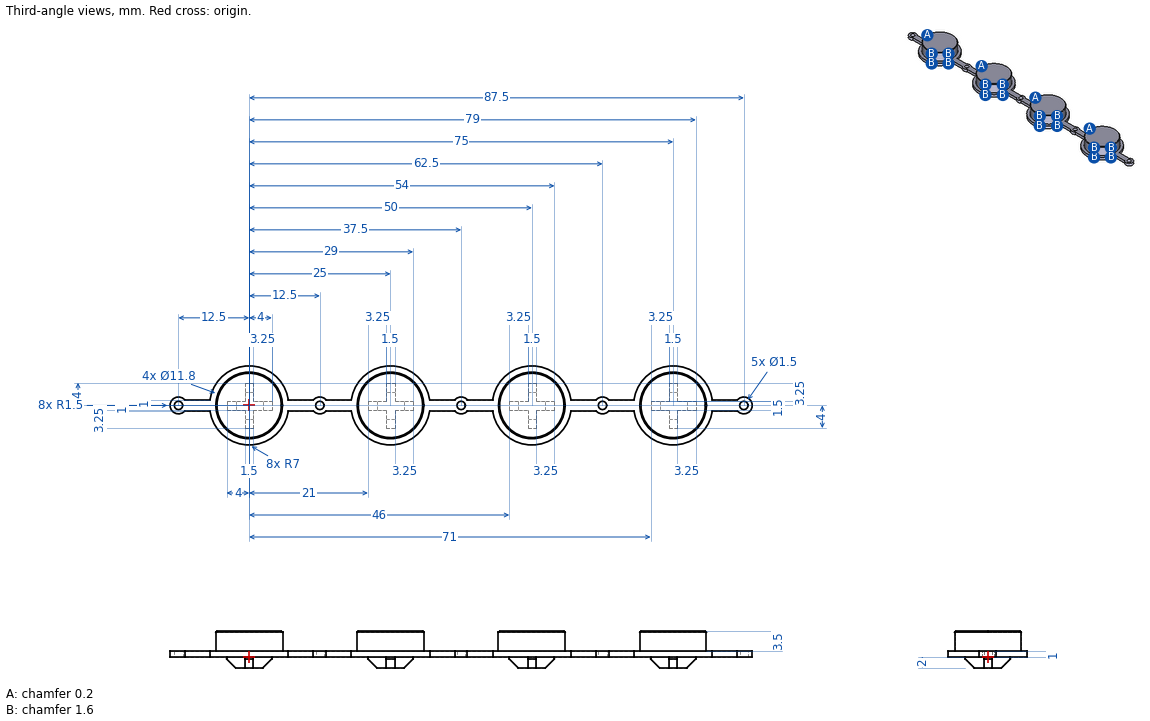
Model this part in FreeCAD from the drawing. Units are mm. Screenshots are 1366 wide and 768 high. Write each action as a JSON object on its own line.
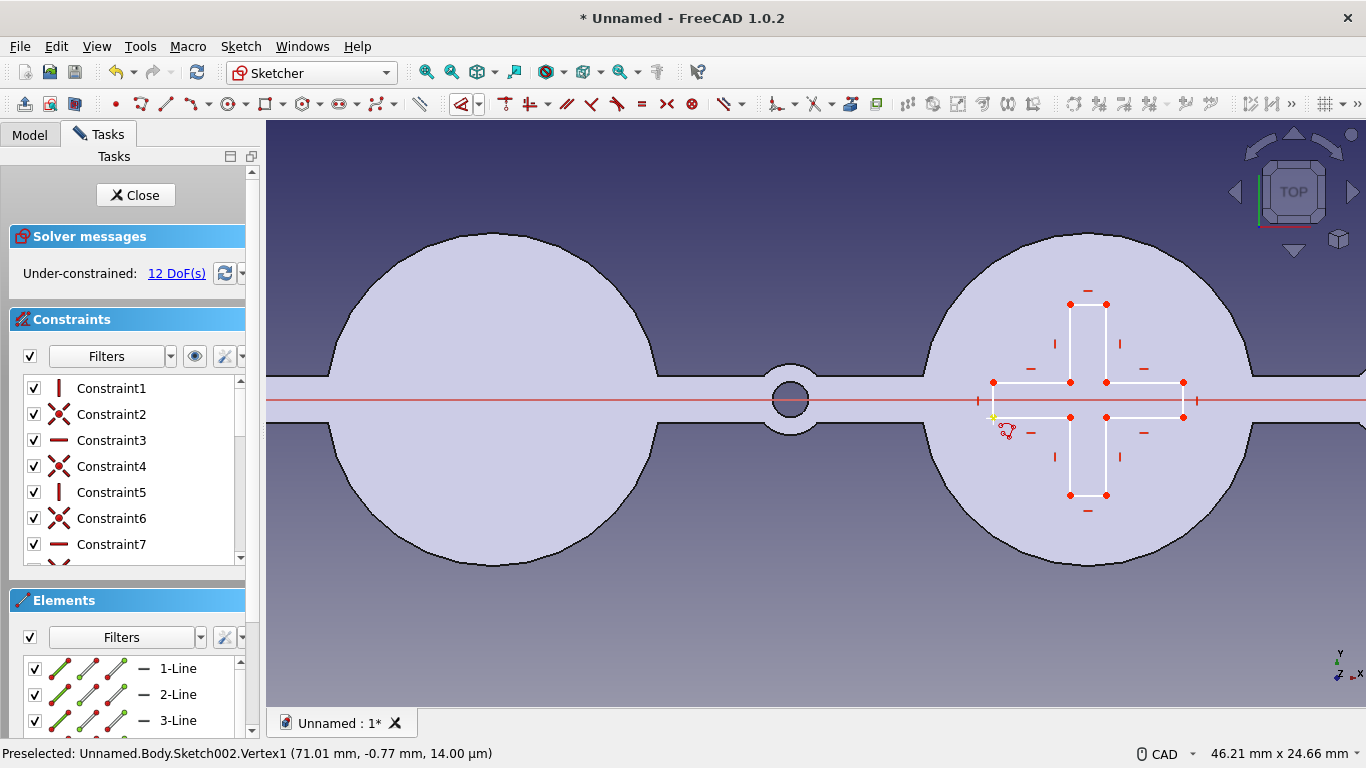
{"action": "left_click", "coordinate": [398, 417]}
{"action": "left_click", "coordinate": [398, 382]}
{"action": "left_click", "coordinate": [475, 382]}
{"action": "left_click", "coordinate": [475, 304]}
{"action": "left_click", "coordinate": [511, 304]}
{"action": "left_click", "coordinate": [511, 382]}
{"action": "left_click", "coordinate": [588, 382]}
{"action": "left_click", "coordinate": [588, 417]}
{"action": "left_click", "coordinate": [511, 417]}
{"action": "left_click", "coordinate": [511, 495]}
{"action": "left_click", "coordinate": [475, 495]}
{"action": "left_click", "coordinate": [475, 417]}
{"action": "left_click", "coordinate": [398, 418]}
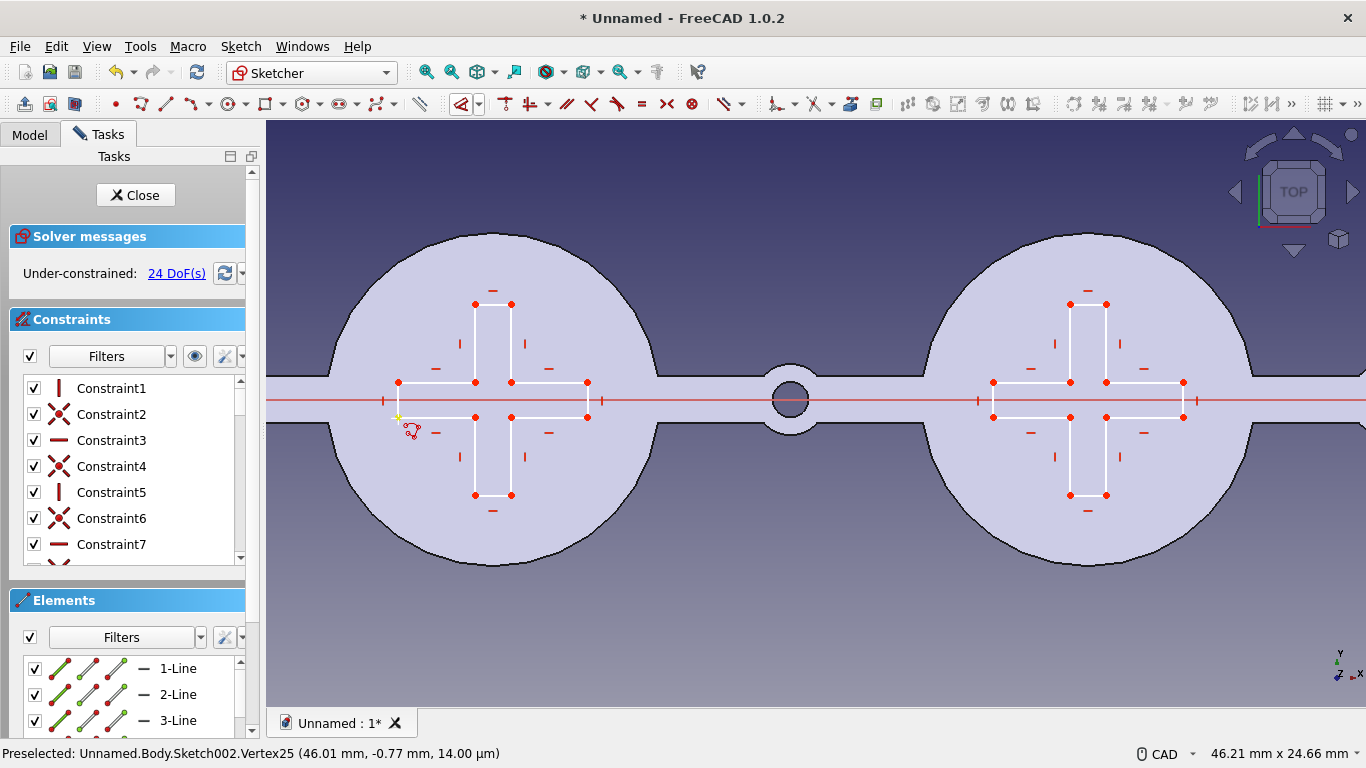
{"action": "scroll", "coordinate": [985, 420], "scroll_direction": "down", "scroll_amount": 6}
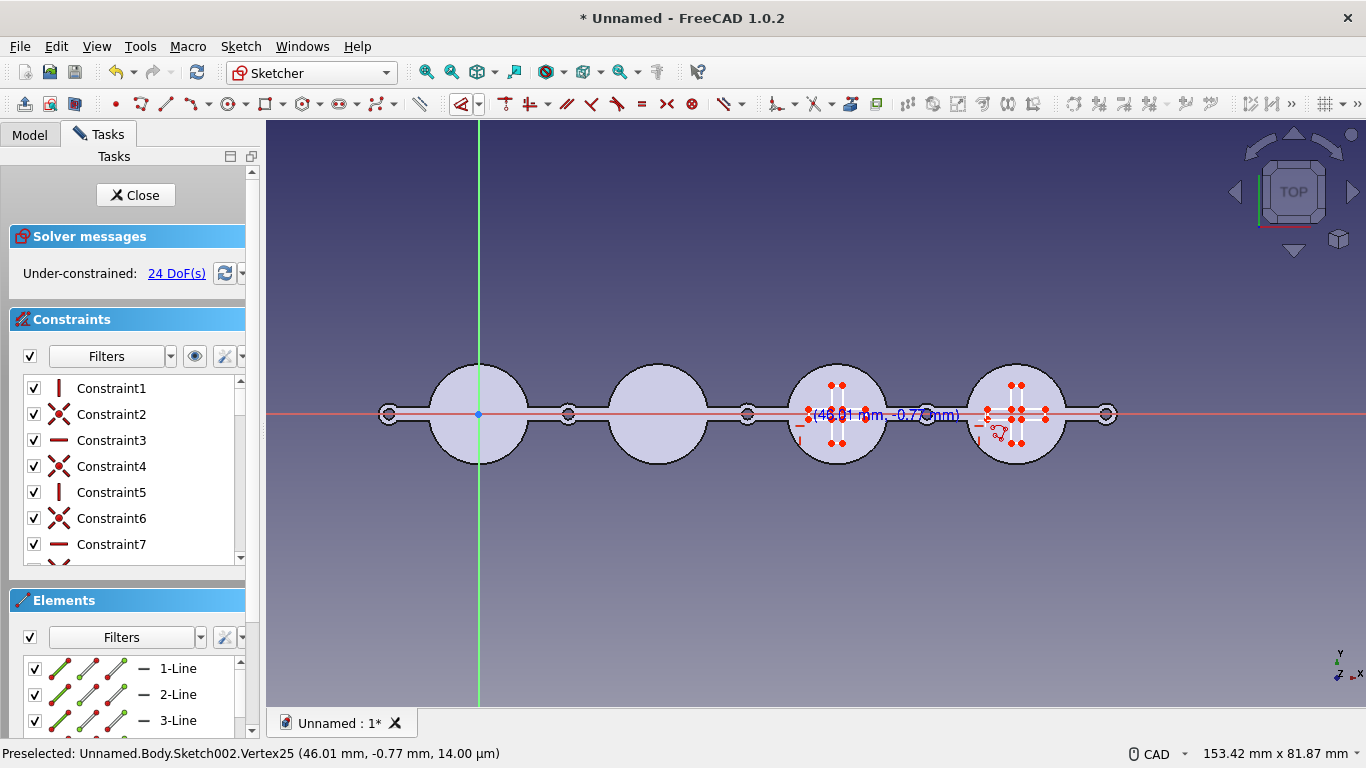
{"action": "scroll", "coordinate": [629, 420], "scroll_direction": "up", "scroll_amount": 6}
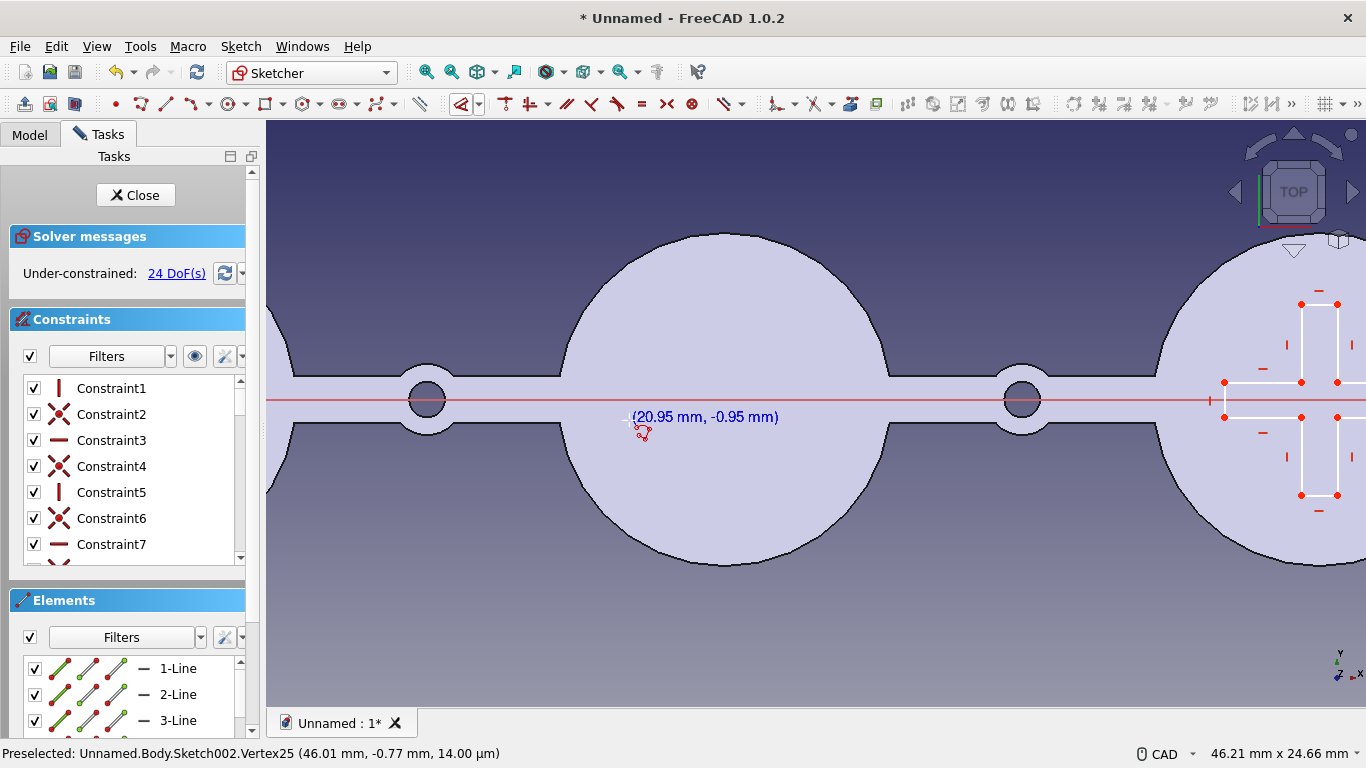
{"action": "left_click", "coordinate": [629, 417]}
{"action": "left_click", "coordinate": [629, 382]}
{"action": "left_click", "coordinate": [707, 382]}
{"action": "left_click", "coordinate": [707, 304]}
{"action": "left_click", "coordinate": [742, 304]}
{"action": "left_click", "coordinate": [742, 382]}
{"action": "left_click", "coordinate": [820, 382]}
{"action": "left_click", "coordinate": [820, 417]}
{"action": "left_click", "coordinate": [742, 417]}
{"action": "left_click", "coordinate": [742, 495]}
{"action": "left_click", "coordinate": [707, 495]}
{"action": "left_click", "coordinate": [707, 417]}
{"action": "left_click", "coordinate": [629, 418]}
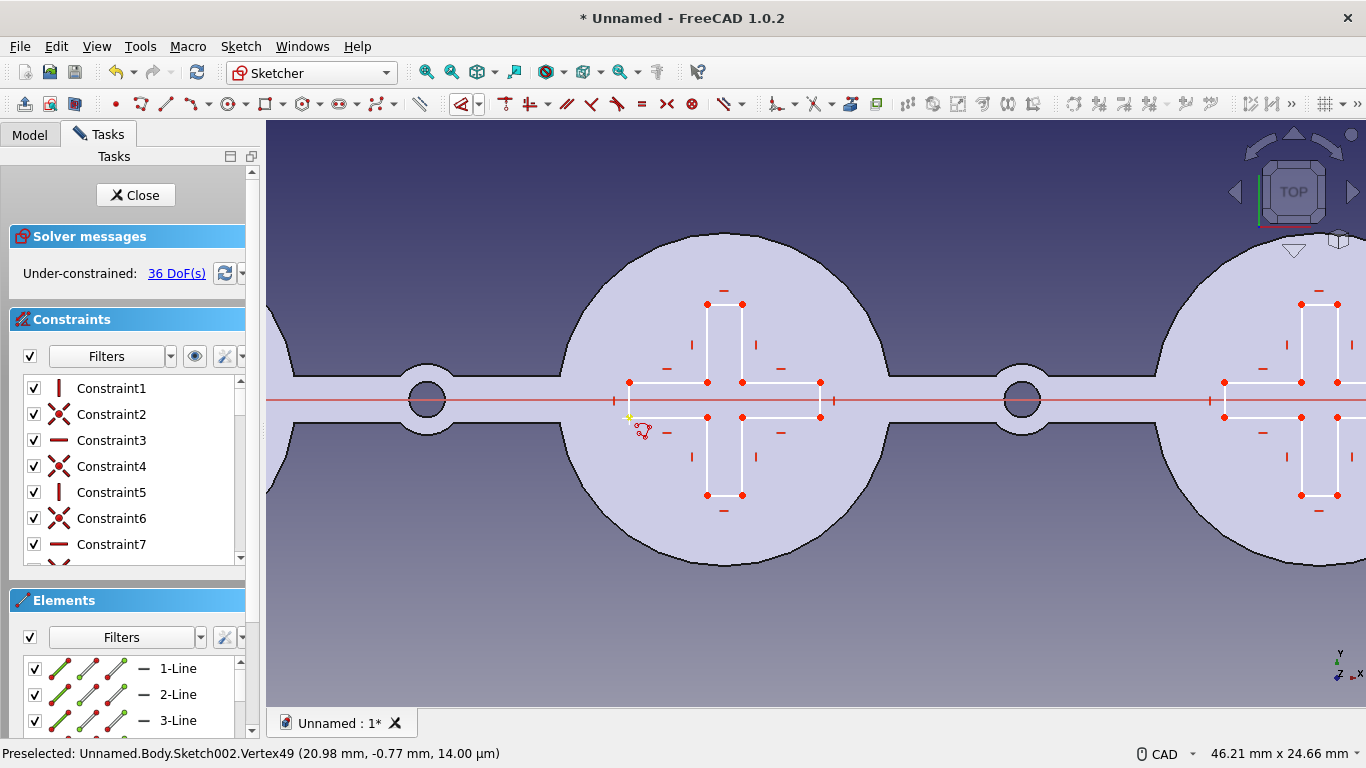
{"action": "scroll", "coordinate": [629, 420], "scroll_direction": "down", "scroll_amount": 6}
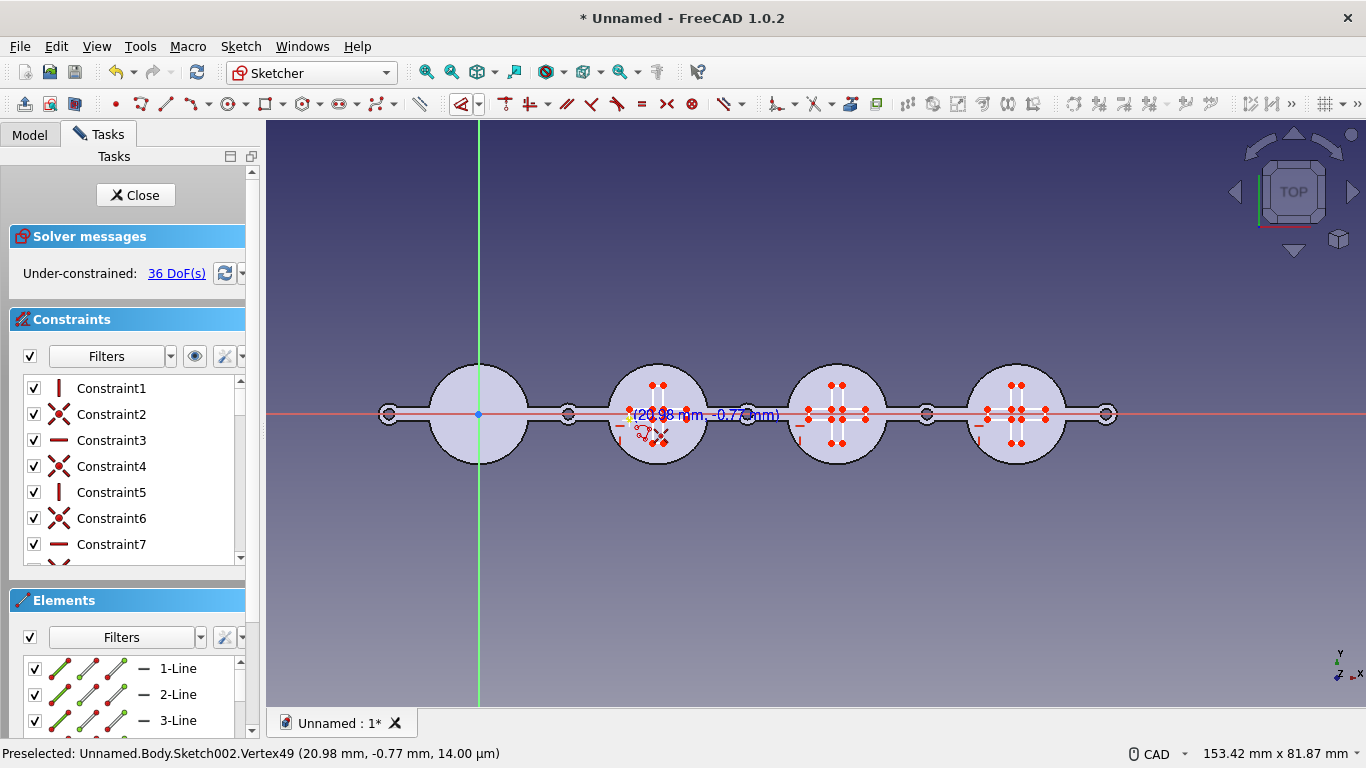
{"action": "scroll", "coordinate": [484, 409], "scroll_direction": "up", "scroll_amount": 6}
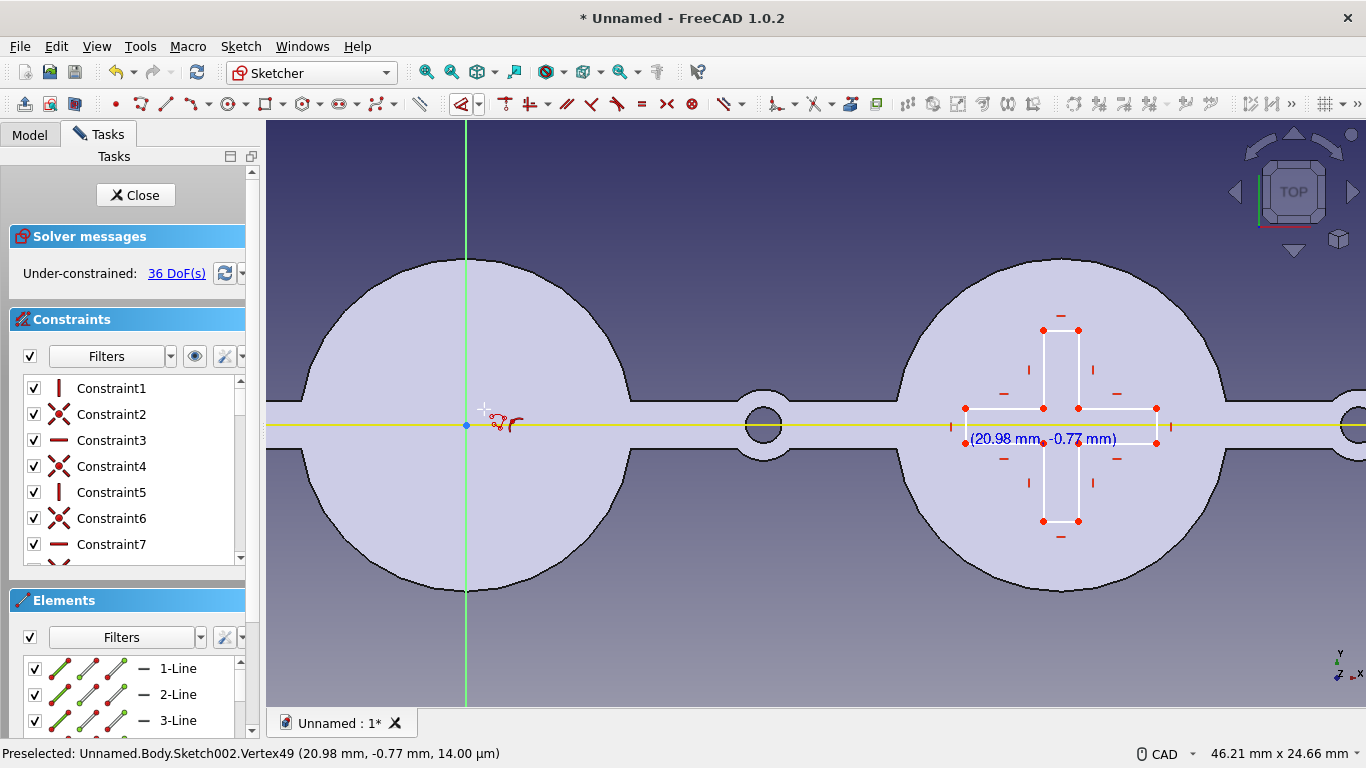
{"action": "left_click", "coordinate": [484, 407]}
{"action": "left_click", "coordinate": [561, 407]}
{"action": "left_click", "coordinate": [561, 443]}
{"action": "left_click", "coordinate": [484, 443]}
{"action": "left_click", "coordinate": [484, 520]}
{"action": "left_click", "coordinate": [448, 520]}
{"action": "left_click", "coordinate": [448, 443]}
{"action": "left_click", "coordinate": [371, 443]}
{"action": "left_click", "coordinate": [371, 407]}
{"action": "left_click", "coordinate": [448, 407]}
{"action": "left_click", "coordinate": [448, 330]}
{"action": "left_click", "coordinate": [484, 330]}
{"action": "left_click", "coordinate": [484, 408]}
{"action": "key", "text": "Escape"}
{"action": "key", "text": "Escape"}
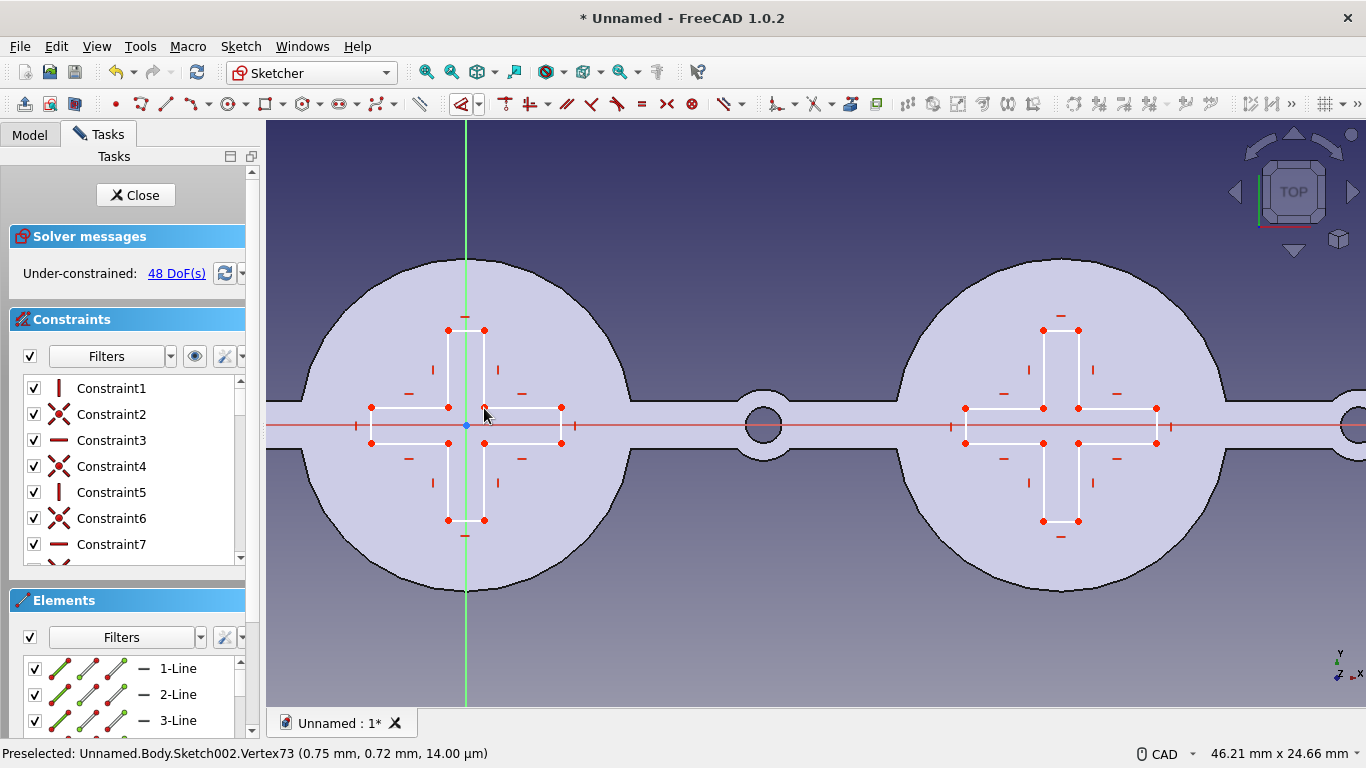
{"action": "scroll", "coordinate": [484, 408], "scroll_direction": "down", "scroll_amount": 6}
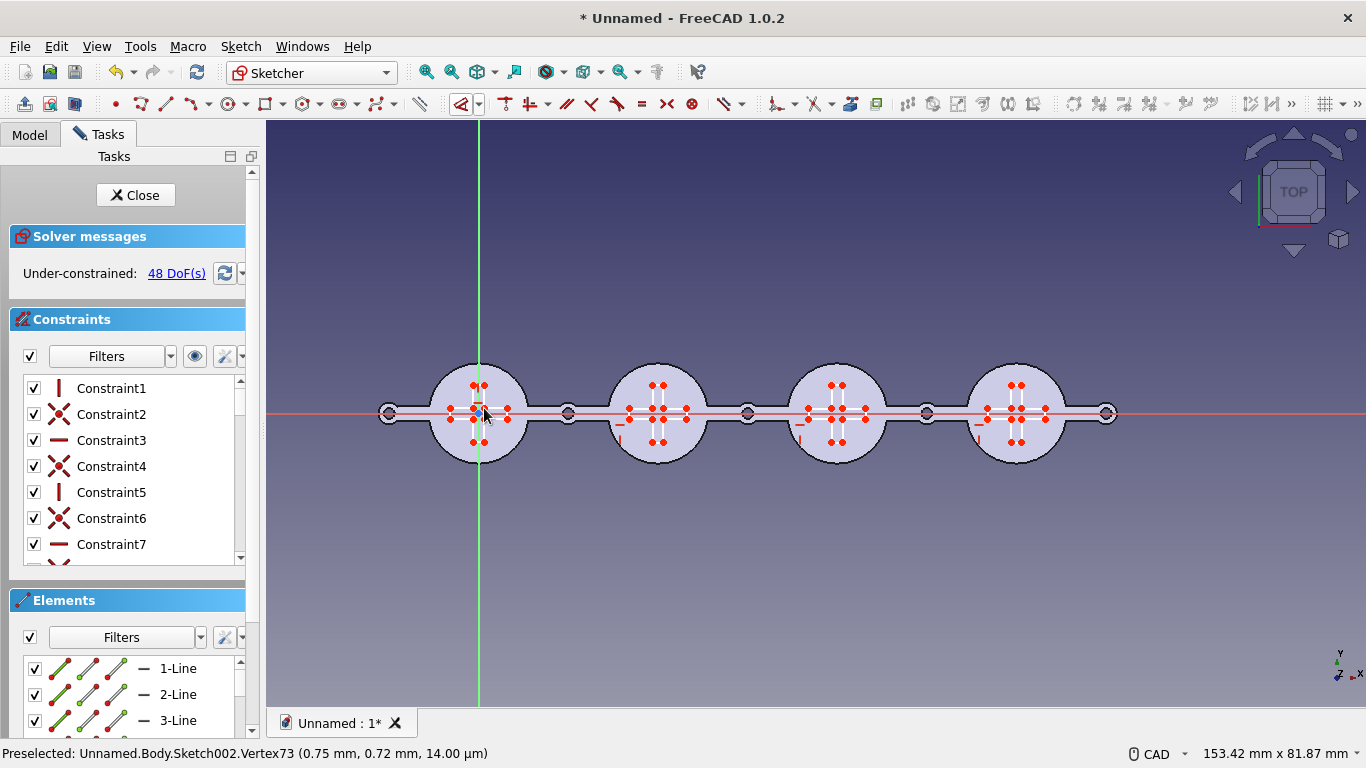
{"action": "scroll", "coordinate": [1011, 385], "scroll_direction": "up", "scroll_amount": 2}